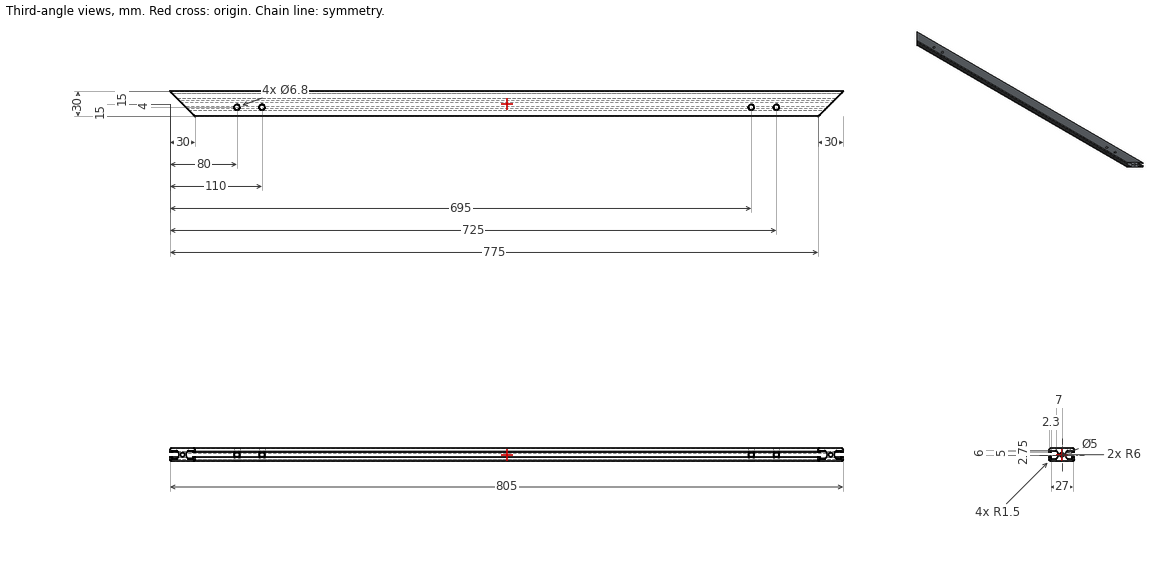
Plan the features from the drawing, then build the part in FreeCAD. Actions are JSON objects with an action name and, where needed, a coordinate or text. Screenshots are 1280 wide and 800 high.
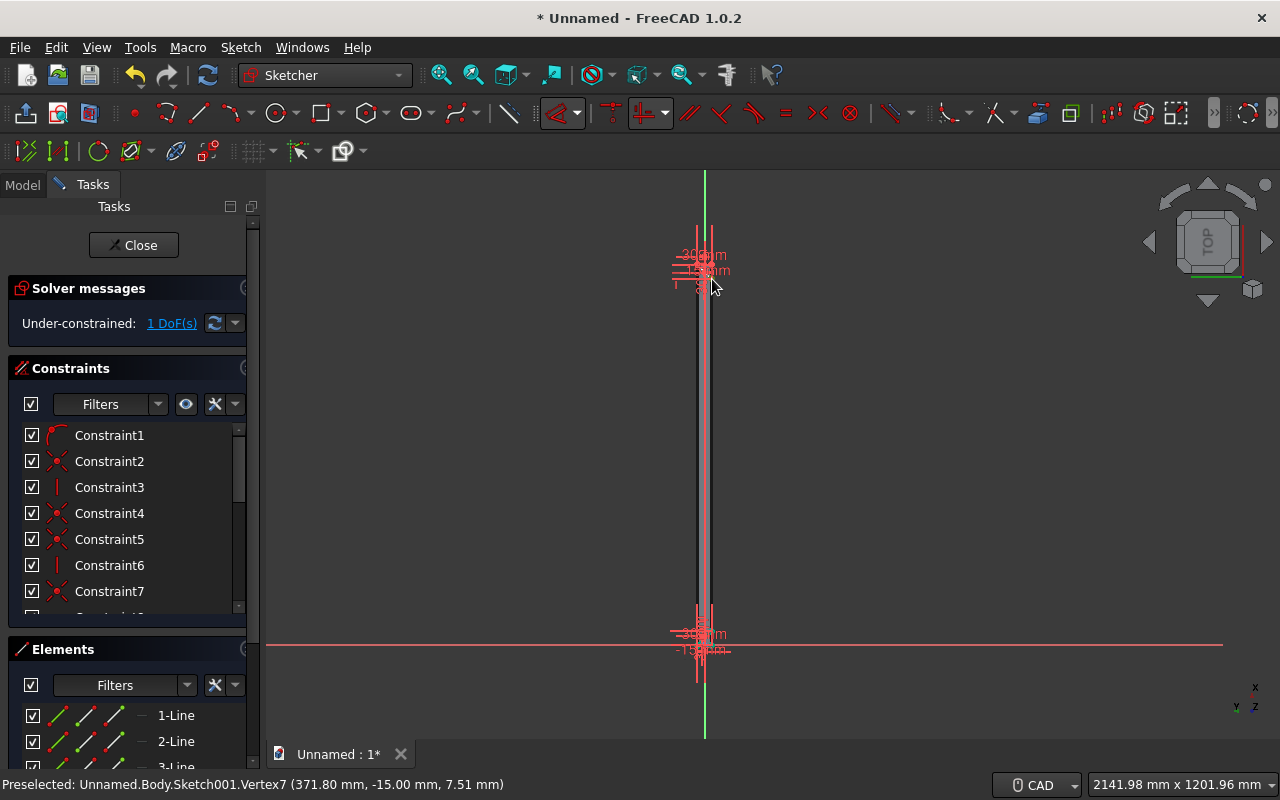
{"action": "left_click", "coordinate": [580, 114]}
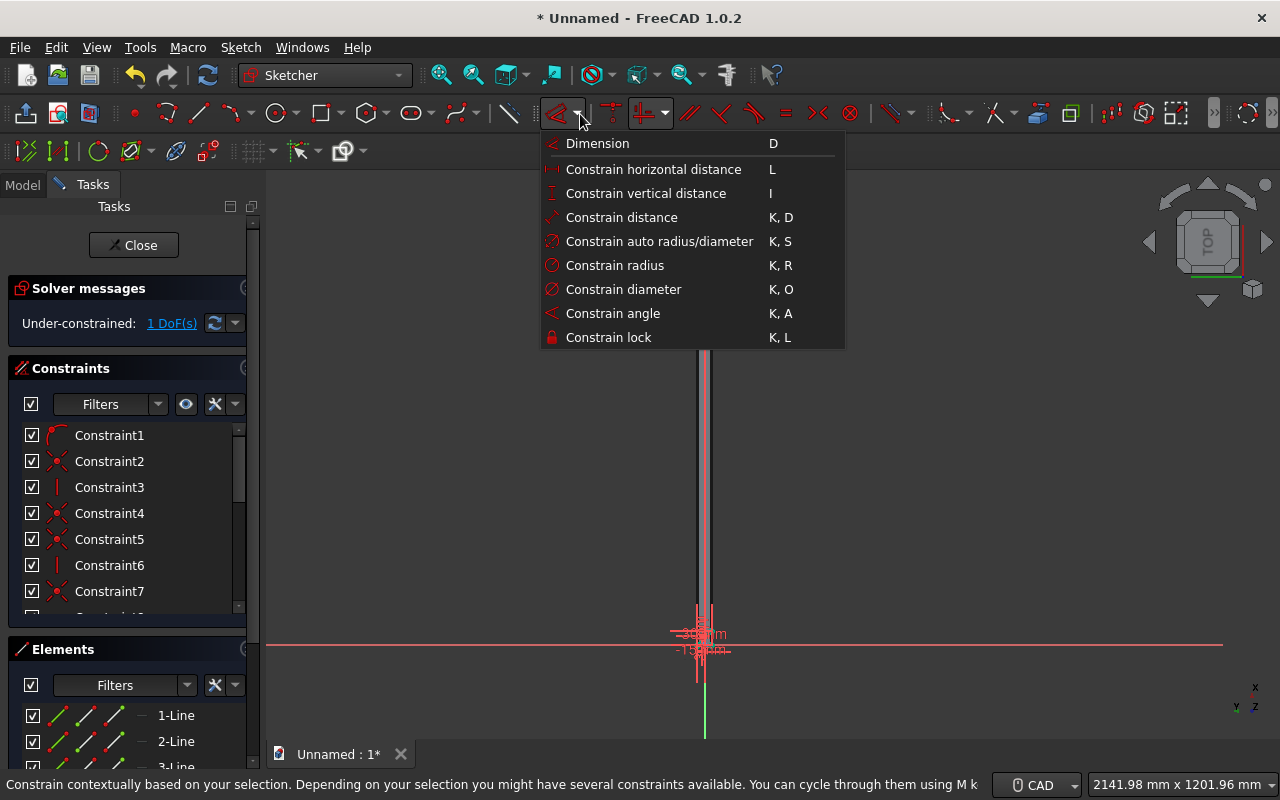
{"action": "left_click", "coordinate": [693, 193]}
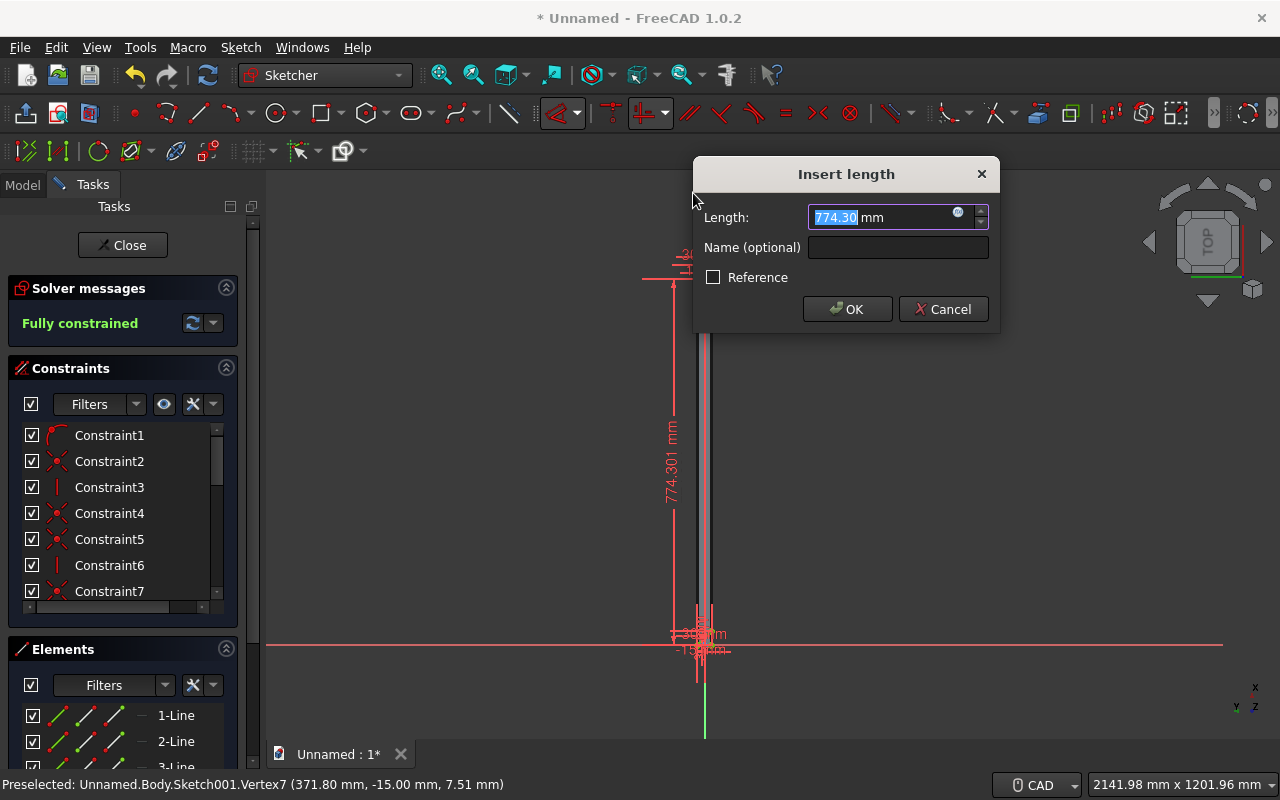
{"action": "type", "text": "775"}
{"action": "key", "text": "Return"}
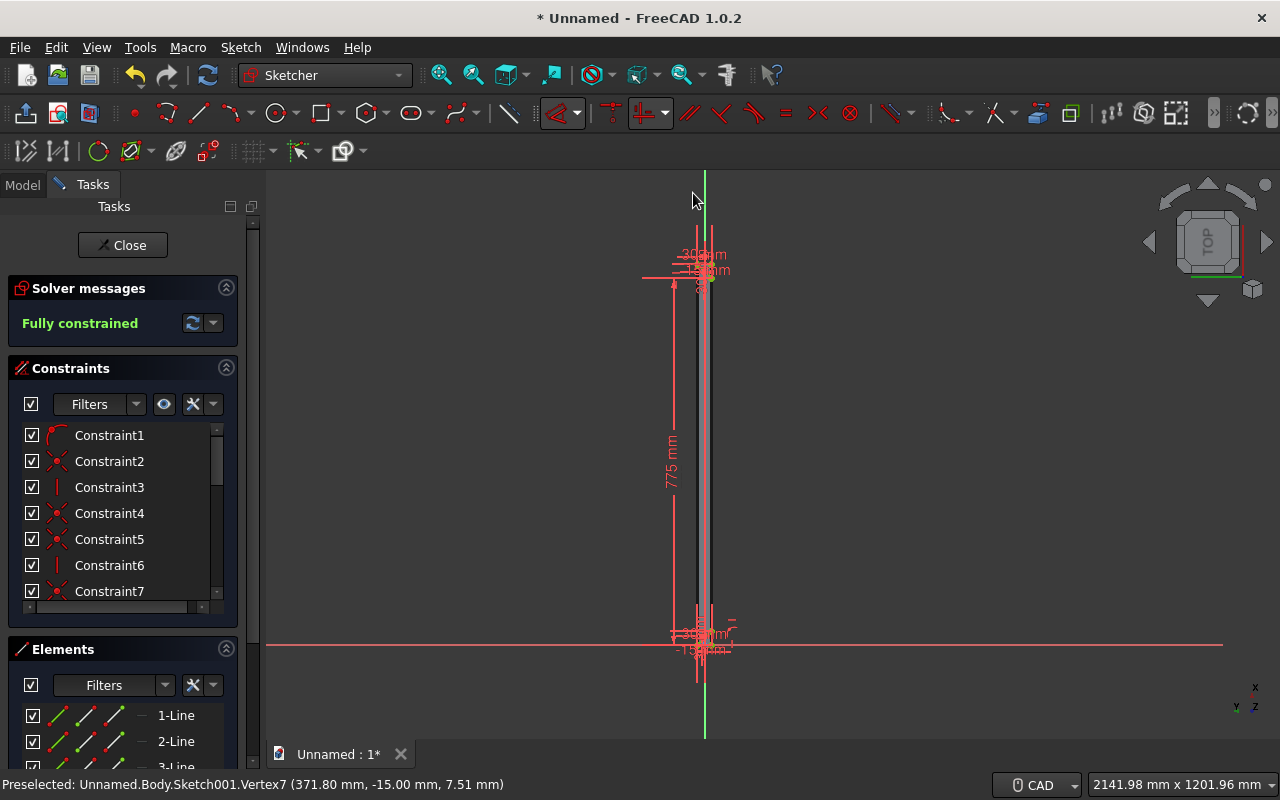
{"action": "left_click", "coordinate": [123, 245]}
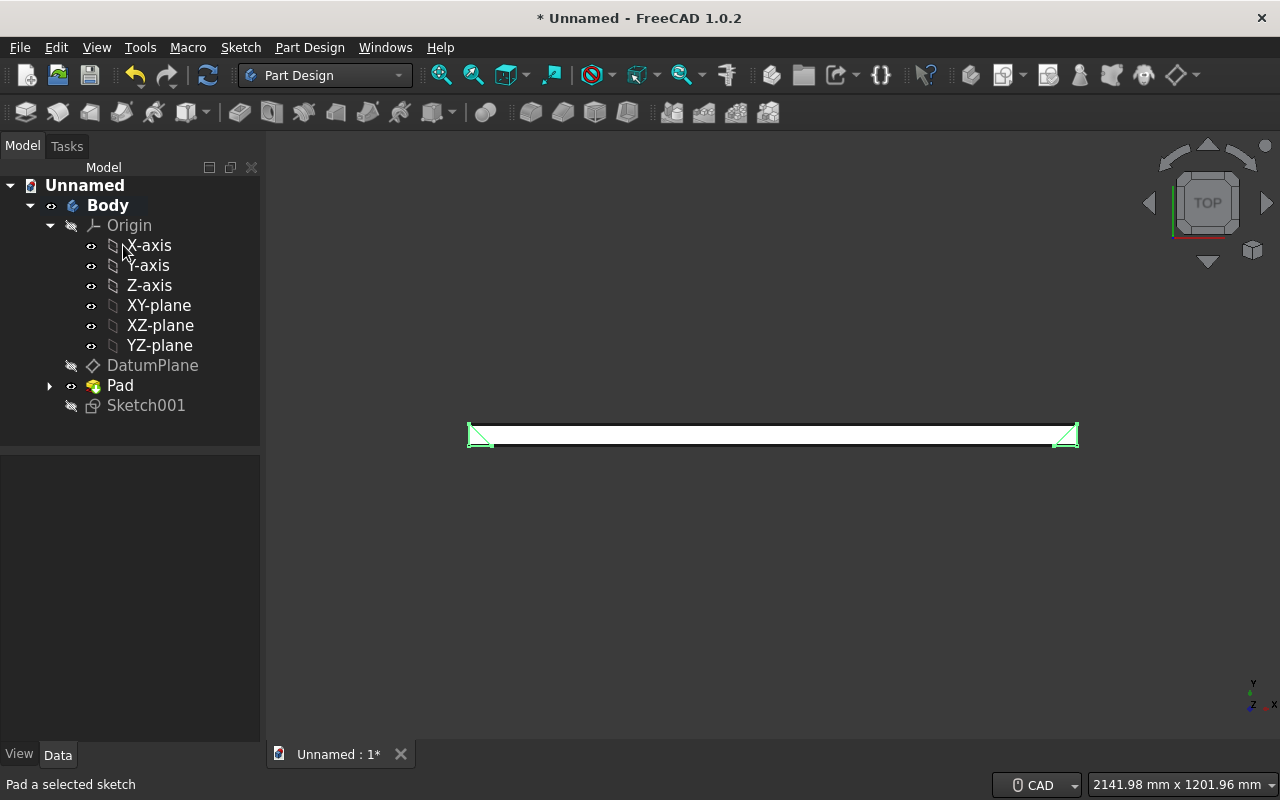
{"action": "left_click", "coordinate": [240, 112]}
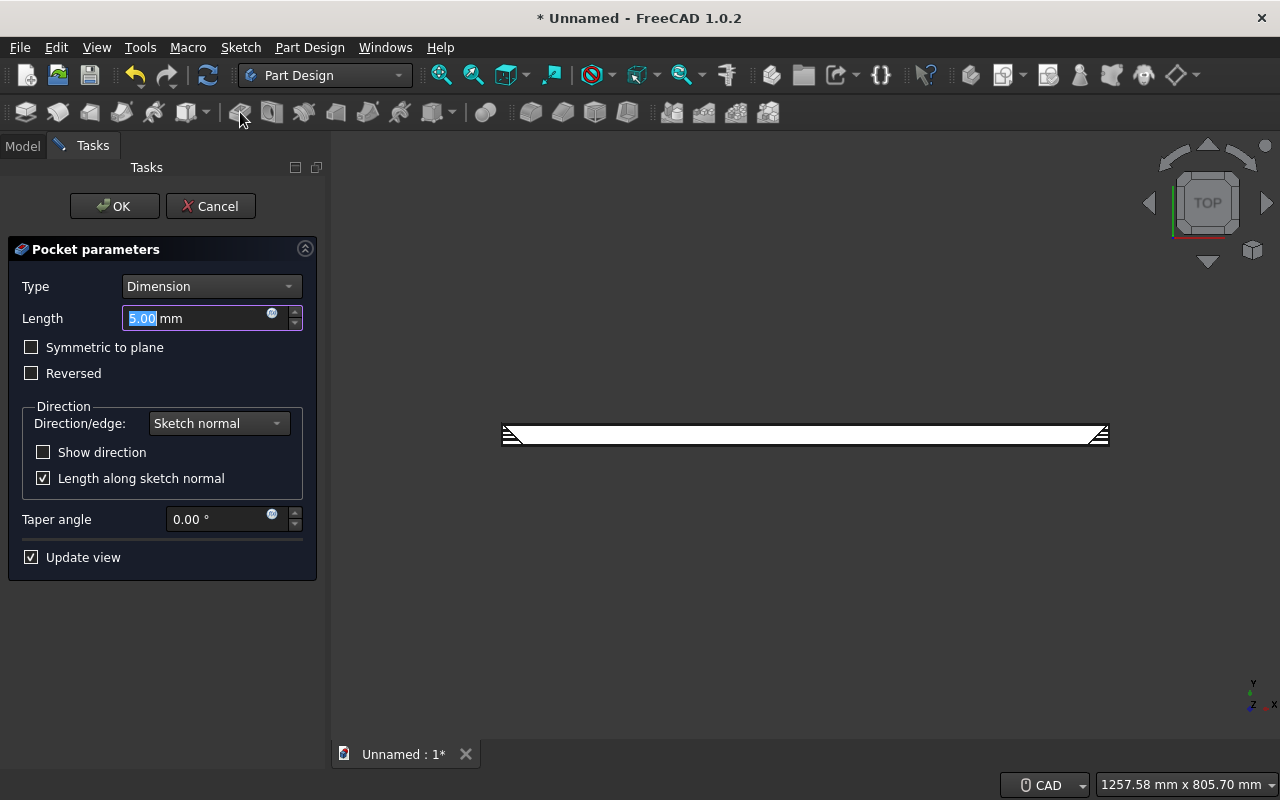
{"action": "left_click", "coordinate": [212, 286]}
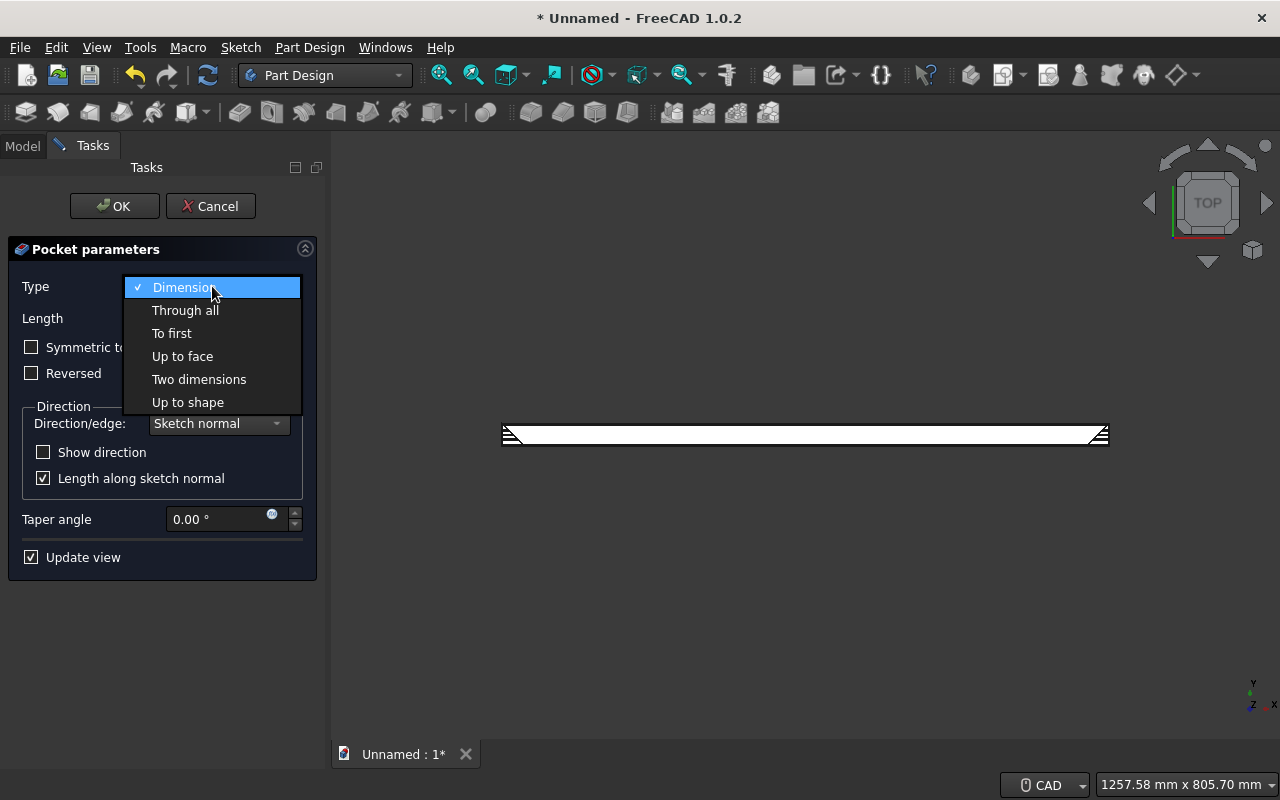
{"action": "left_click", "coordinate": [212, 310]}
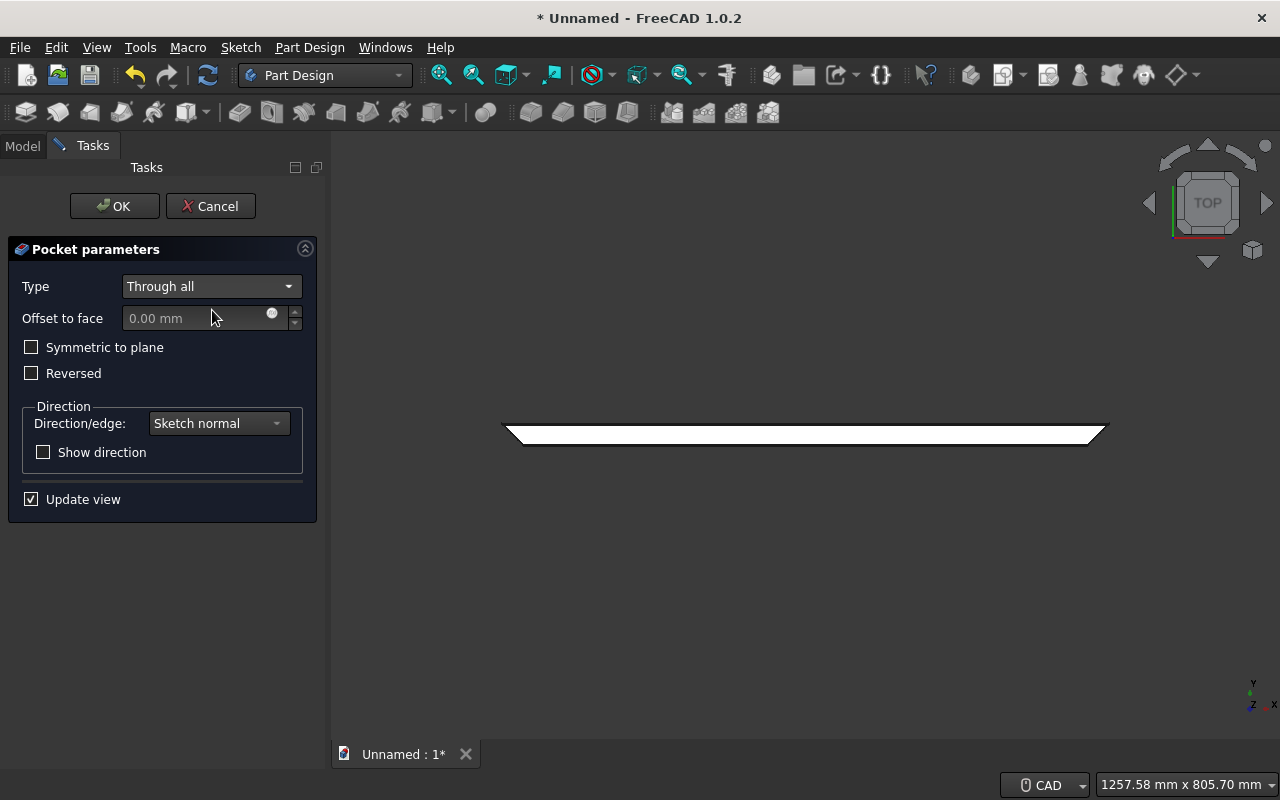
{"action": "left_click", "coordinate": [115, 206]}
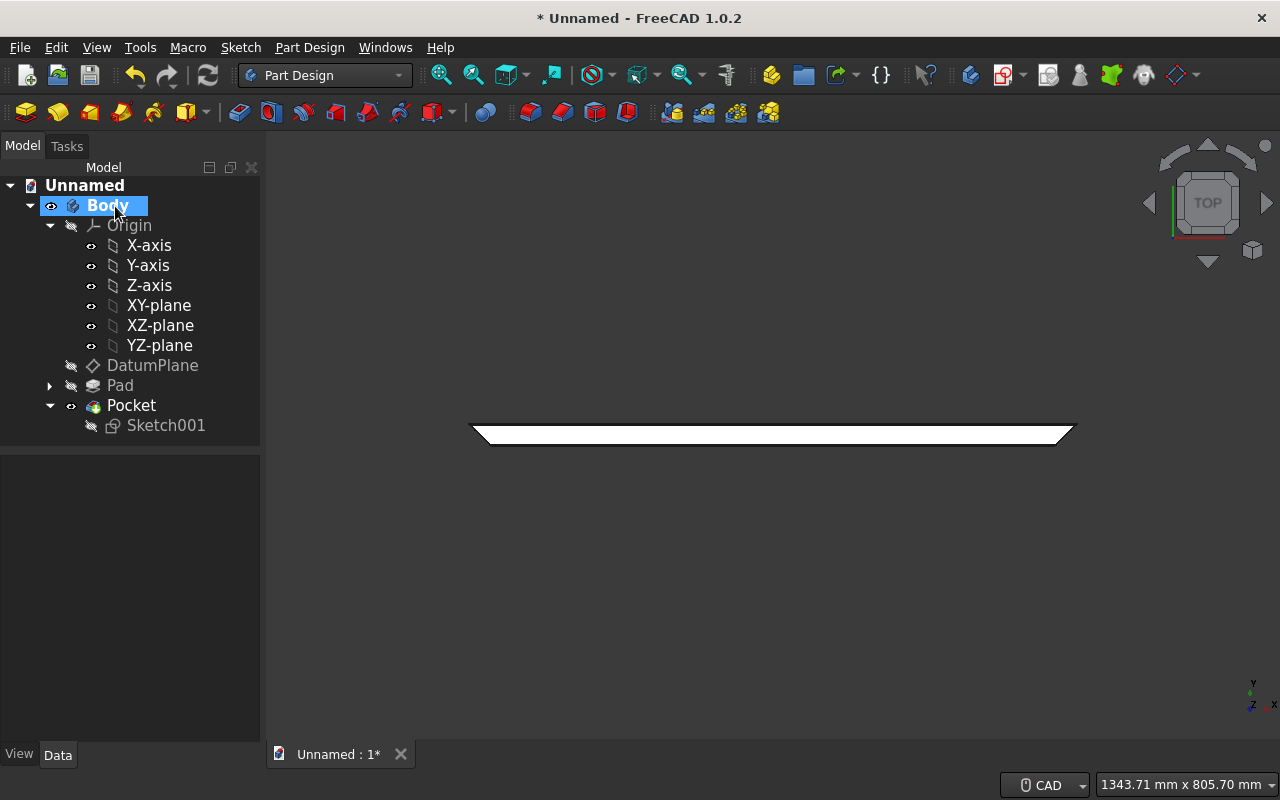
{"action": "left_click", "coordinate": [773, 434]}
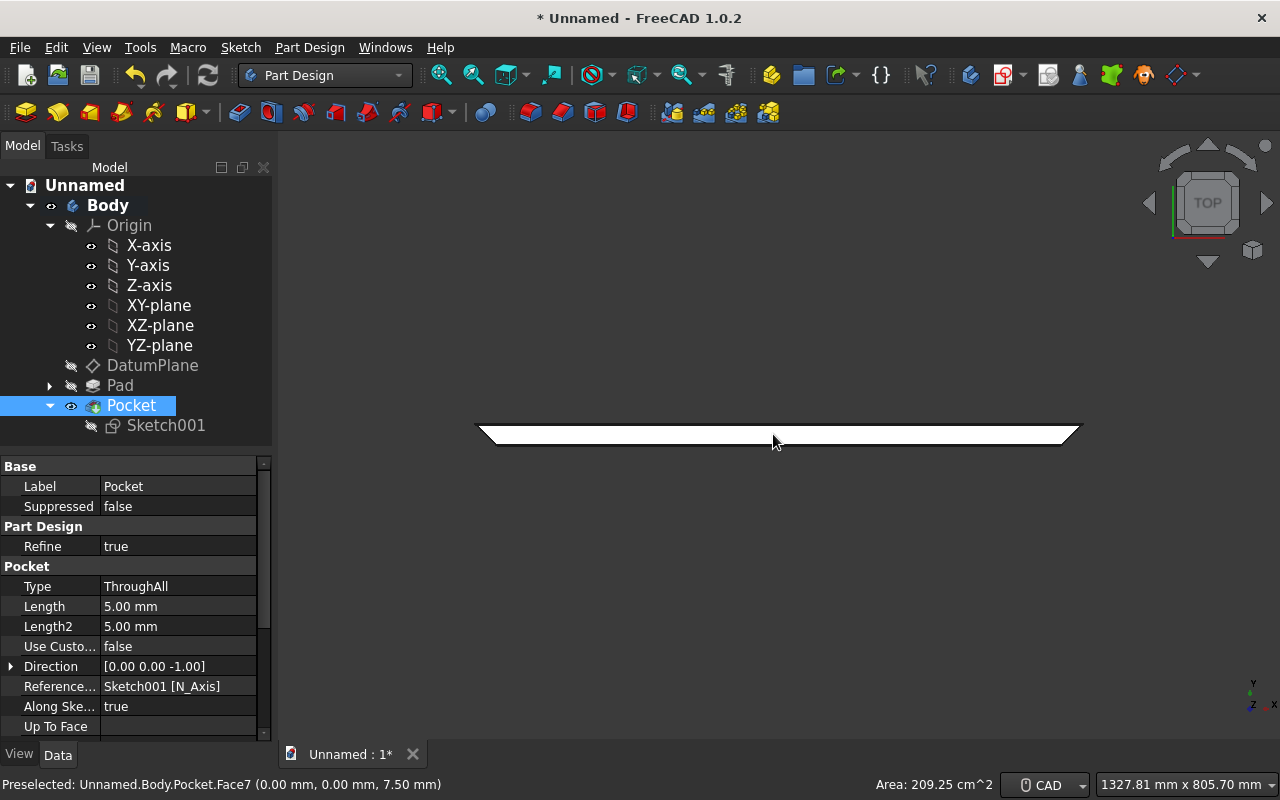
{"action": "left_click", "coordinate": [1004, 76]}